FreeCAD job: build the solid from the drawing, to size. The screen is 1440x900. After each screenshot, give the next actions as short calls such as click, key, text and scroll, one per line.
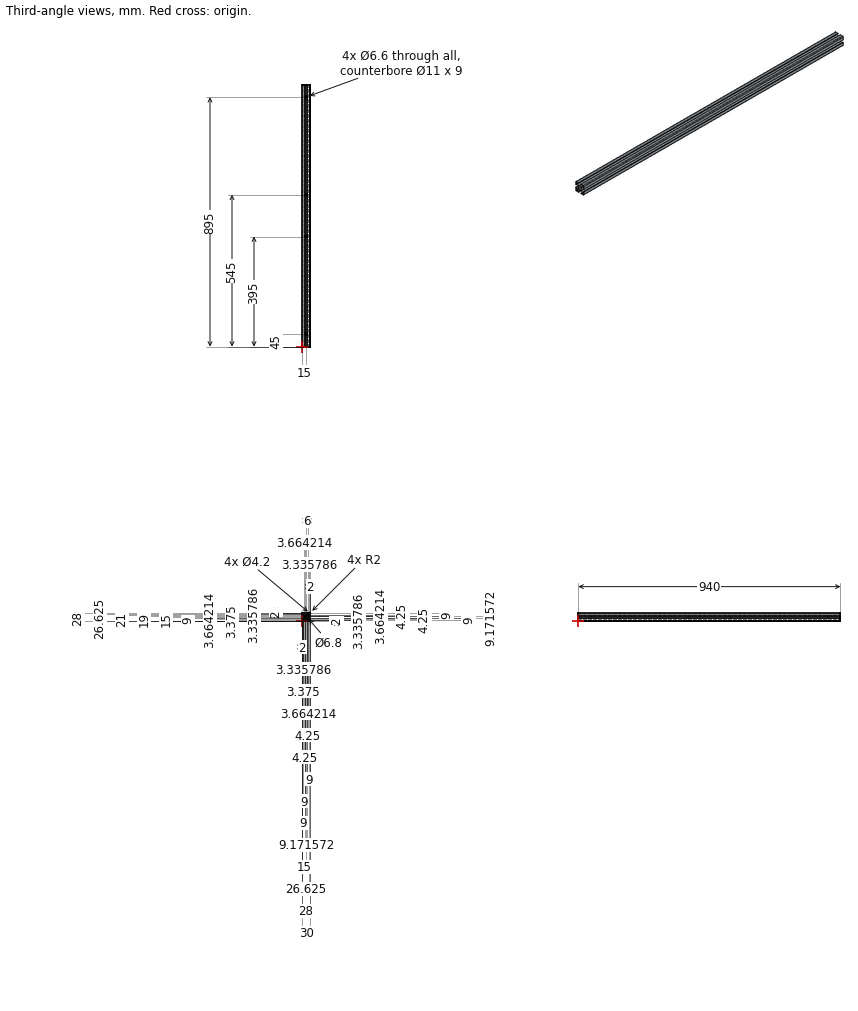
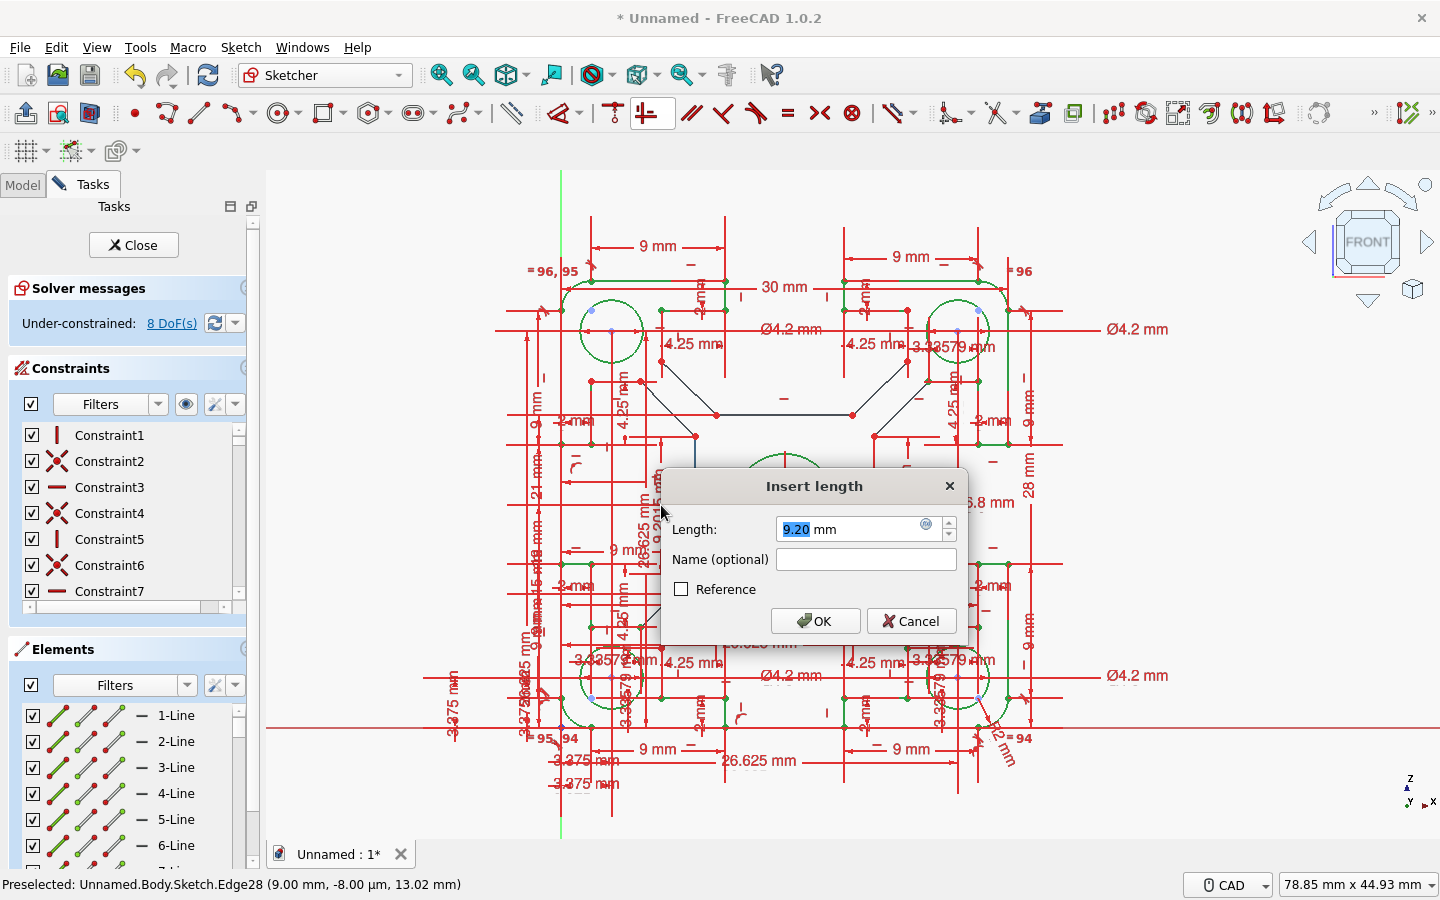
text(9.171572)
key(Return)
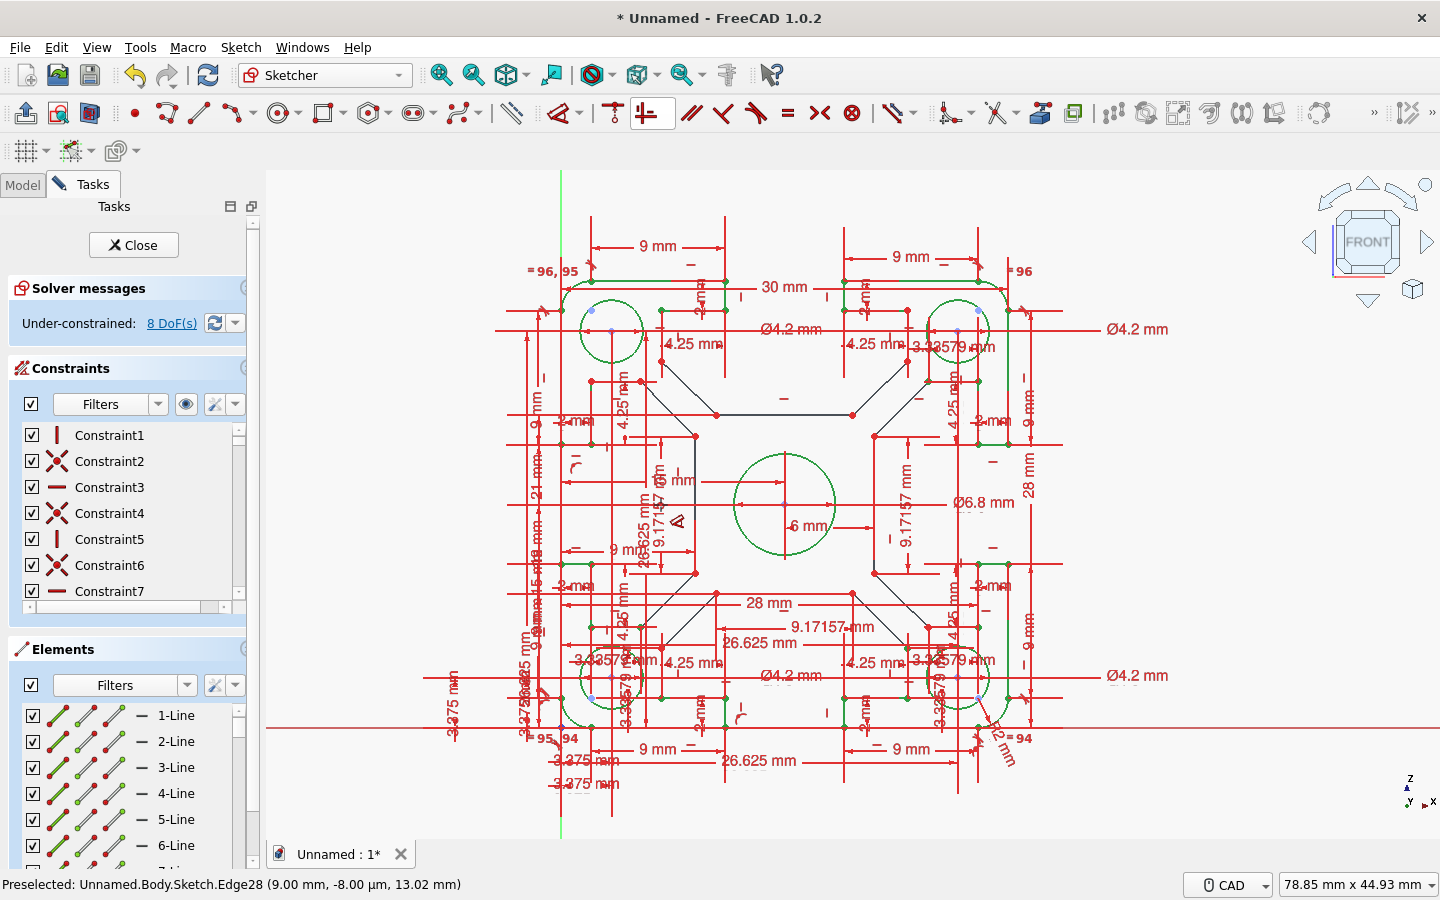
click(626, 382)
click(616, 348)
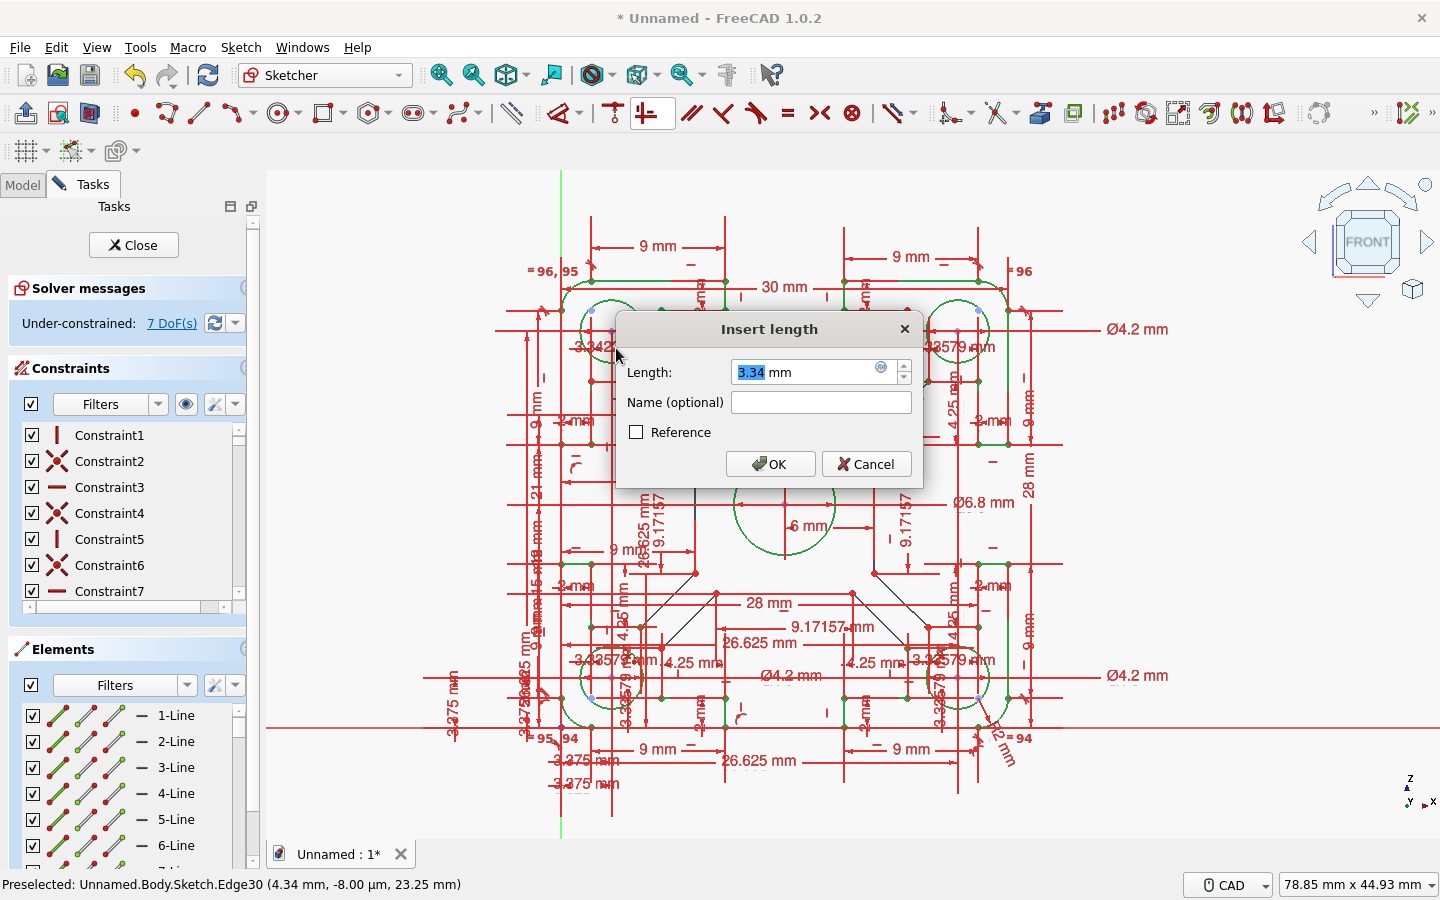
text(3.335786)
key(Return)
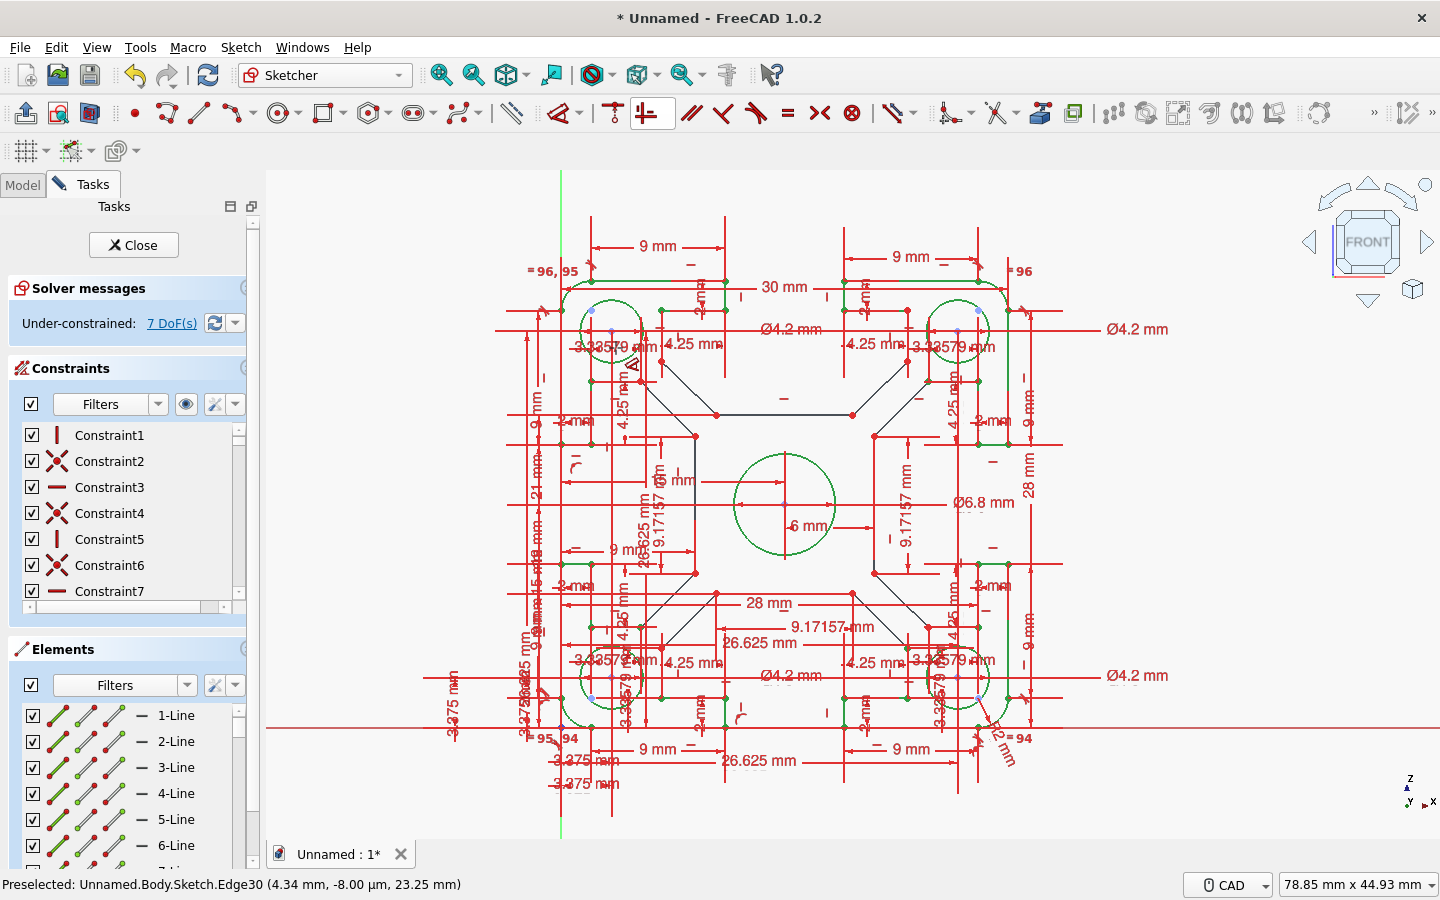
click(662, 326)
click(628, 325)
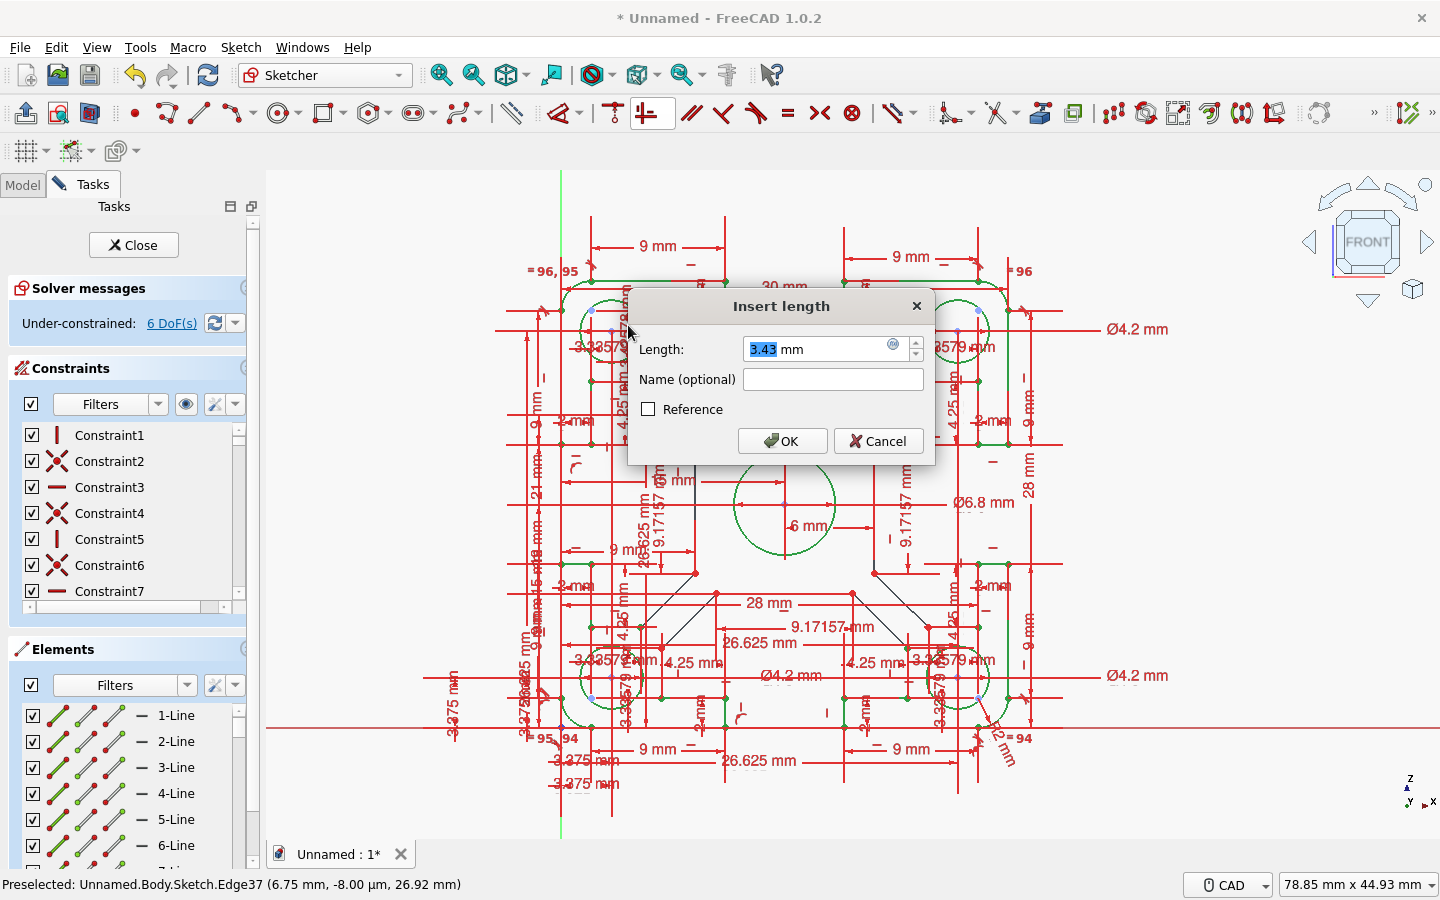
text(3.335786)
key(Return)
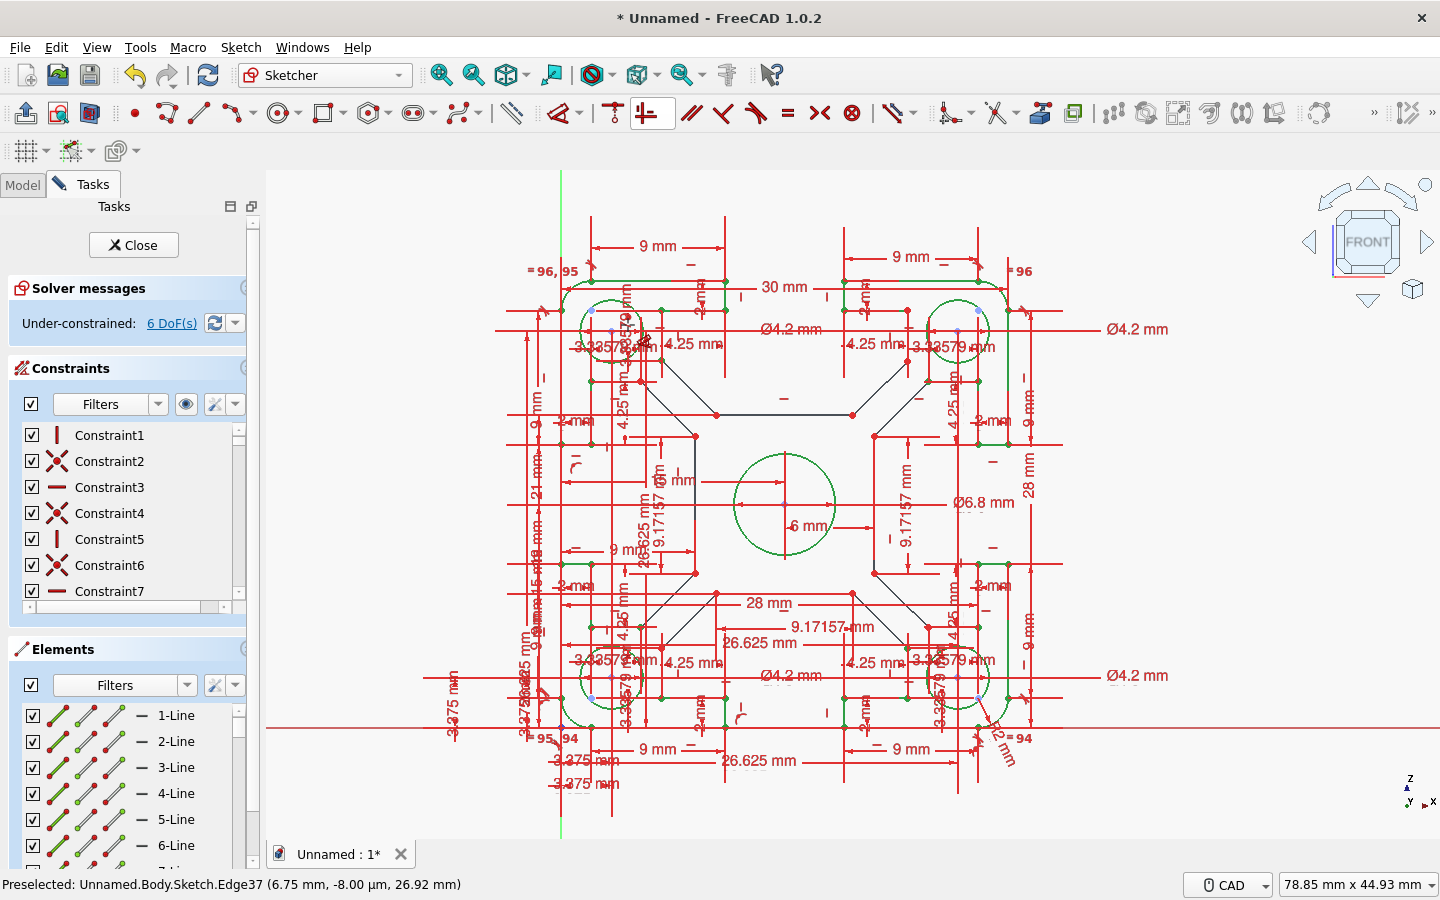
click(758, 415)
click(785, 381)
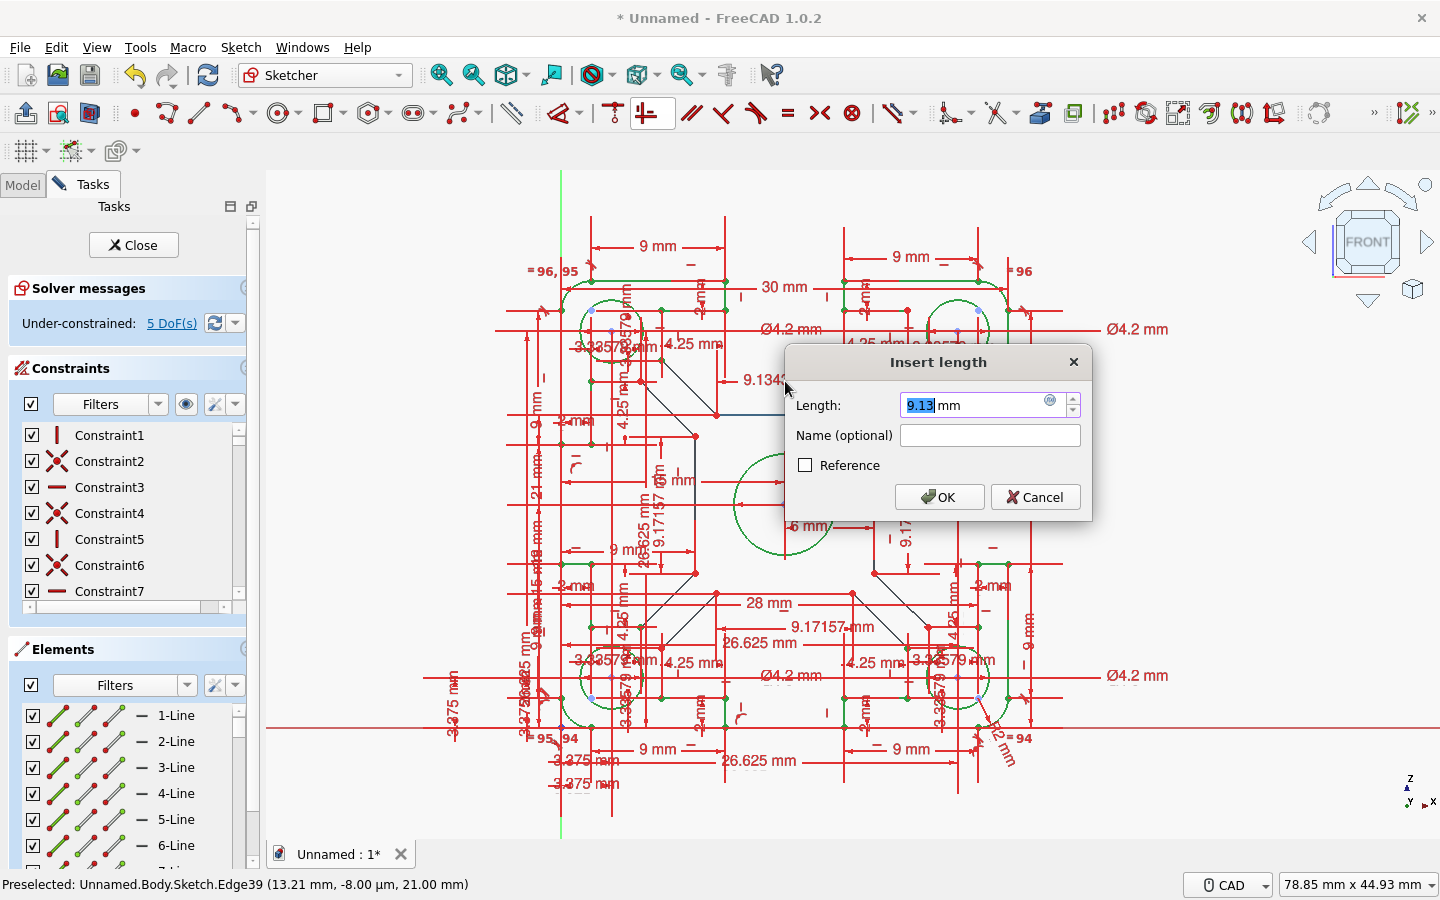
text(9.171572)
key(Return)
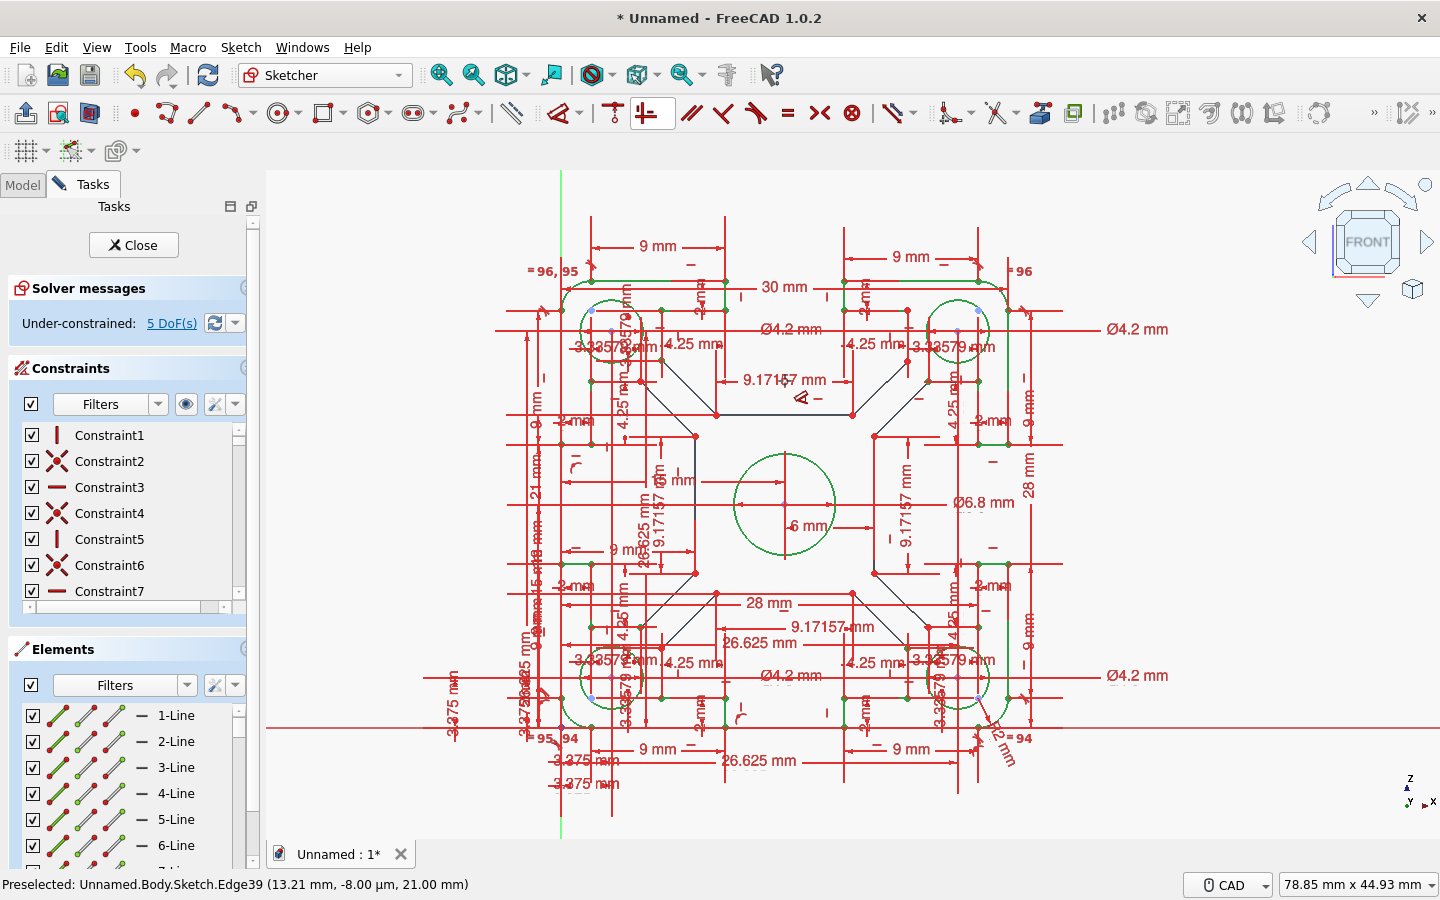
click(908, 347)
click(942, 325)